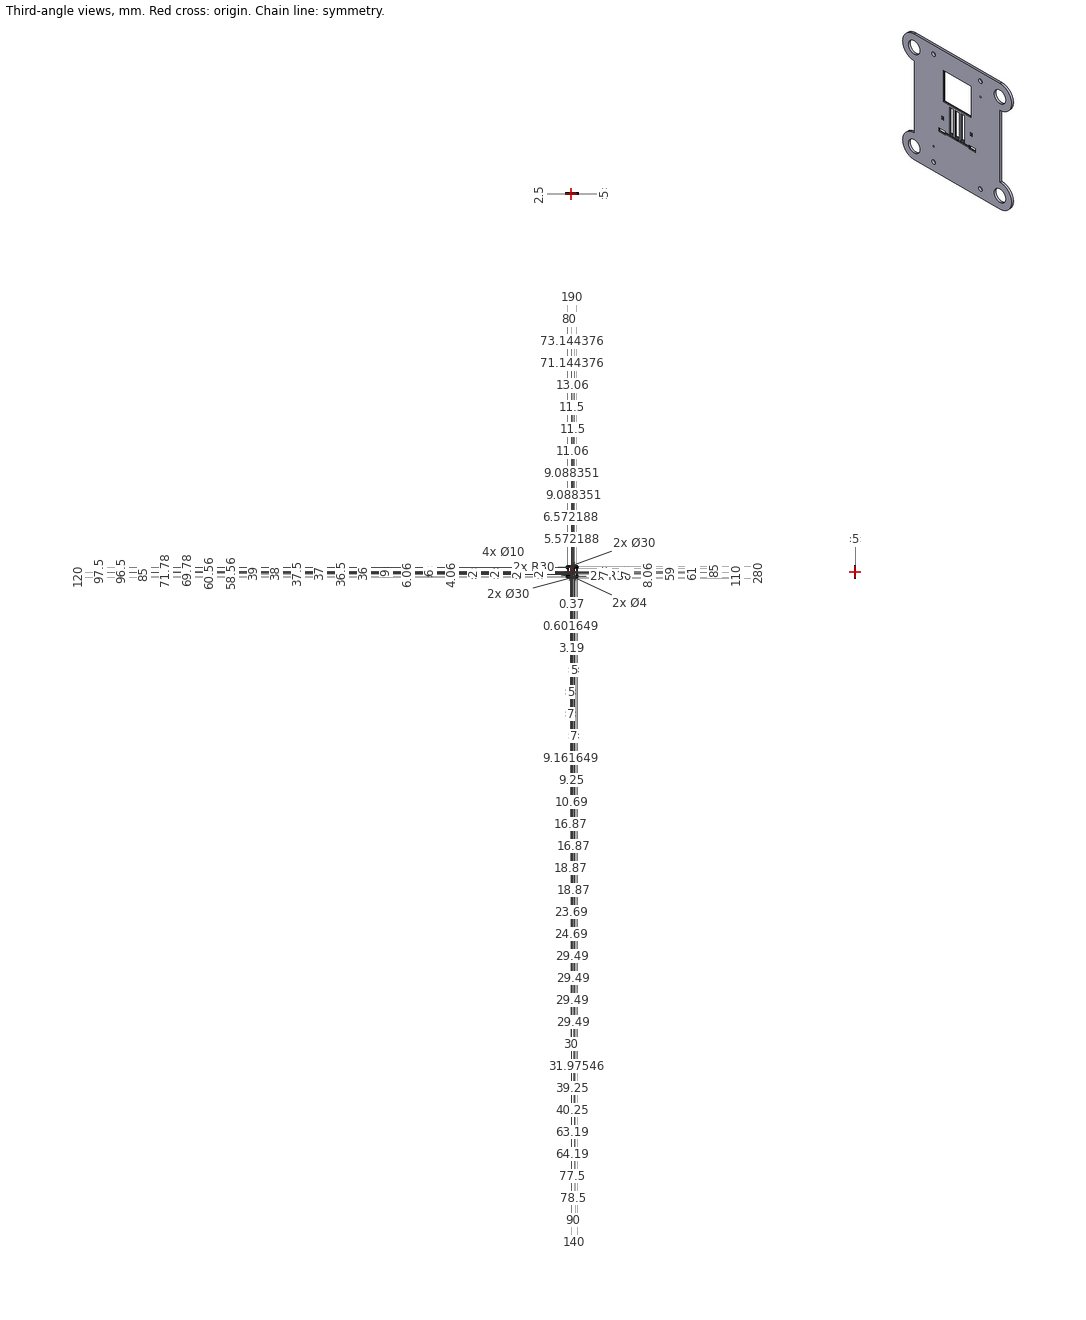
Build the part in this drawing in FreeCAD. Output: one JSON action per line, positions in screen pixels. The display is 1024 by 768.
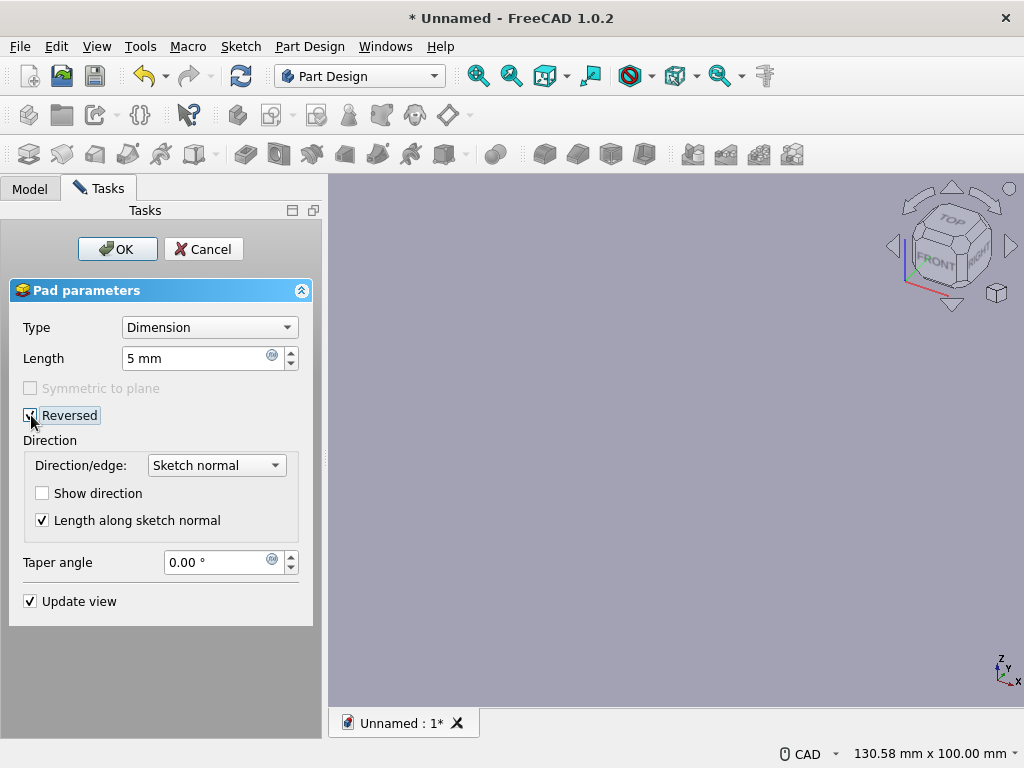
{"action": "left_click", "coordinate": [118, 249]}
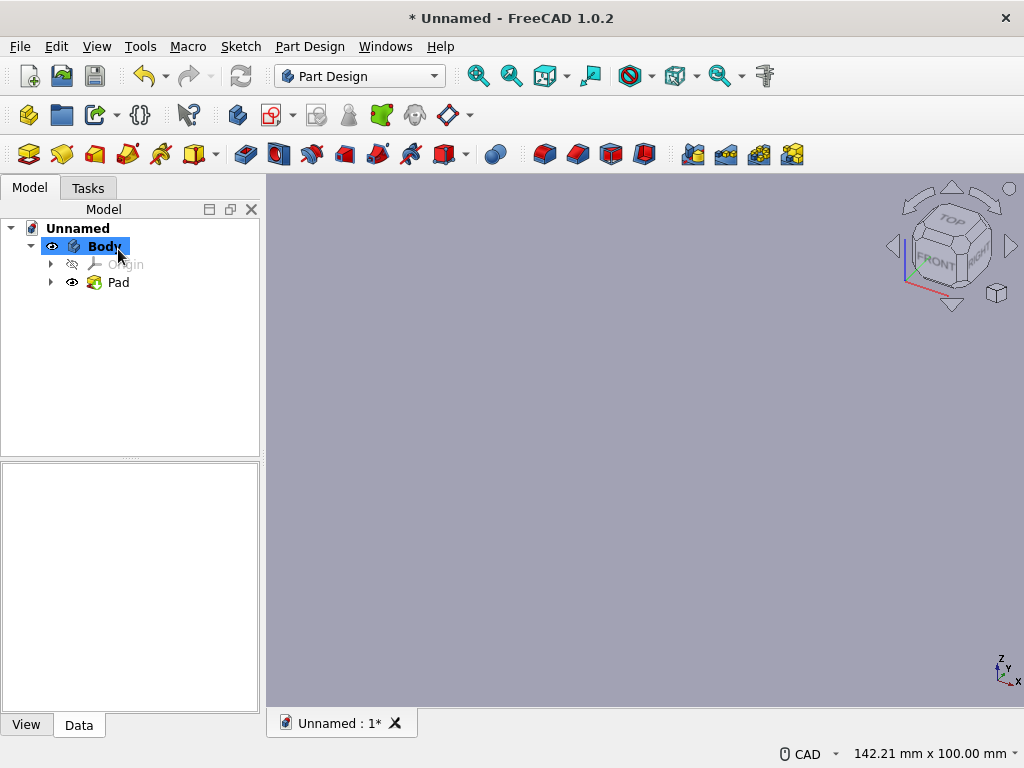
{"action": "left_click", "coordinate": [479, 76]}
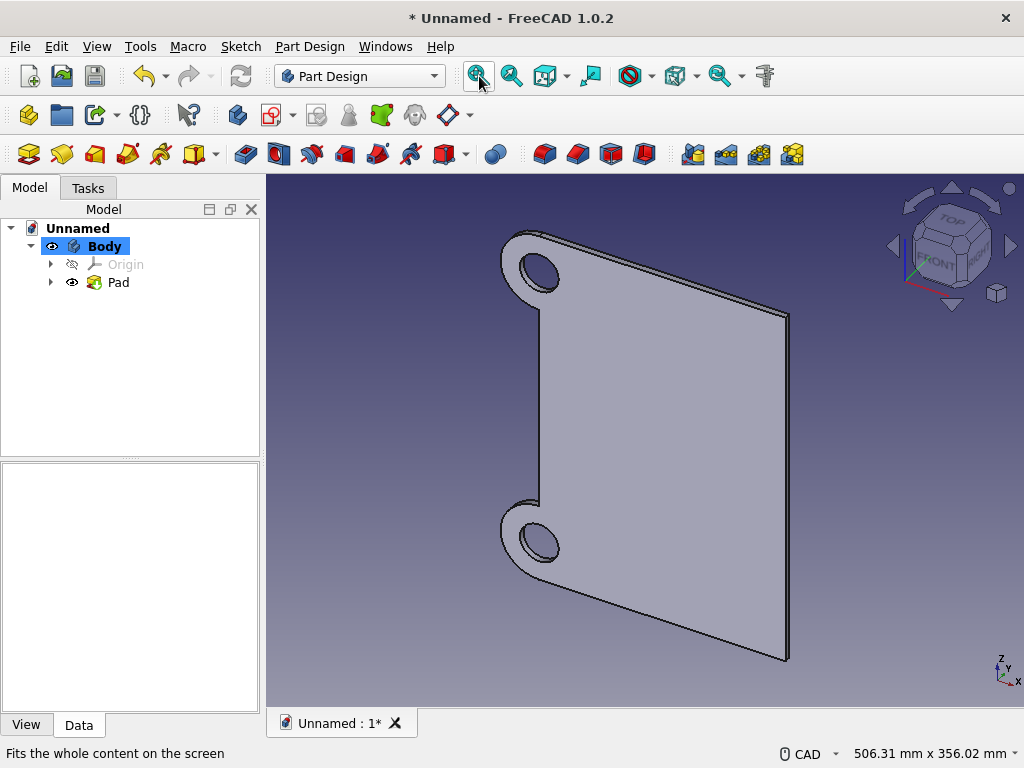
{"action": "key", "text": "4"}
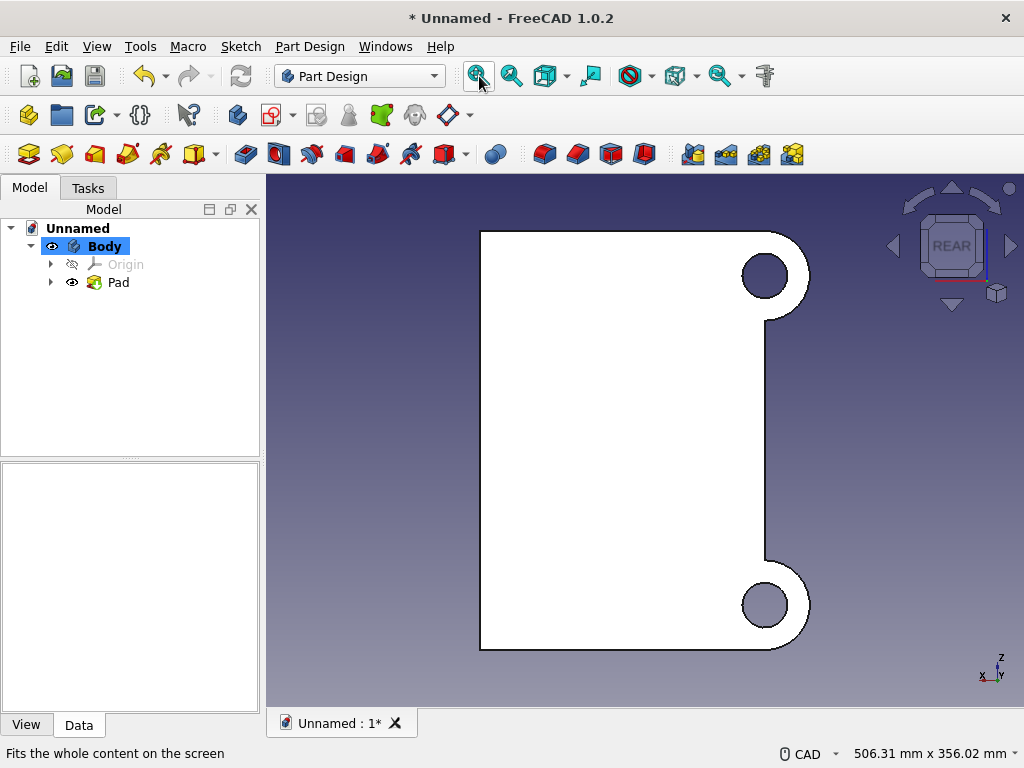
{"action": "left_click", "coordinate": [645, 380]}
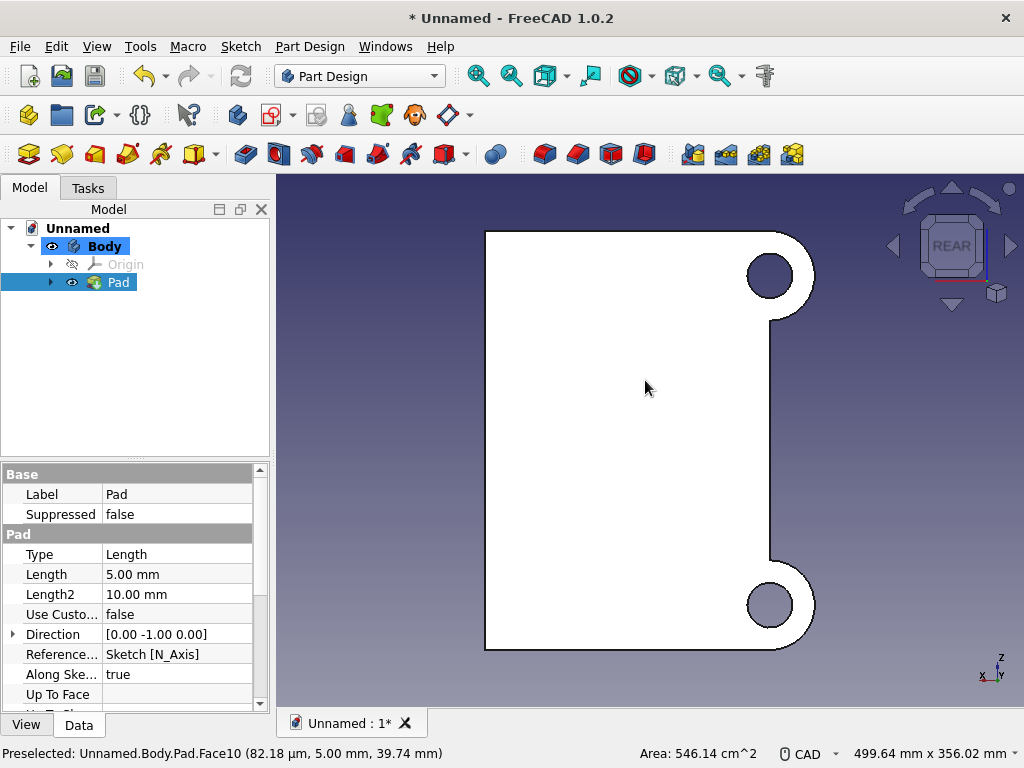
{"action": "left_click", "coordinate": [270, 116]}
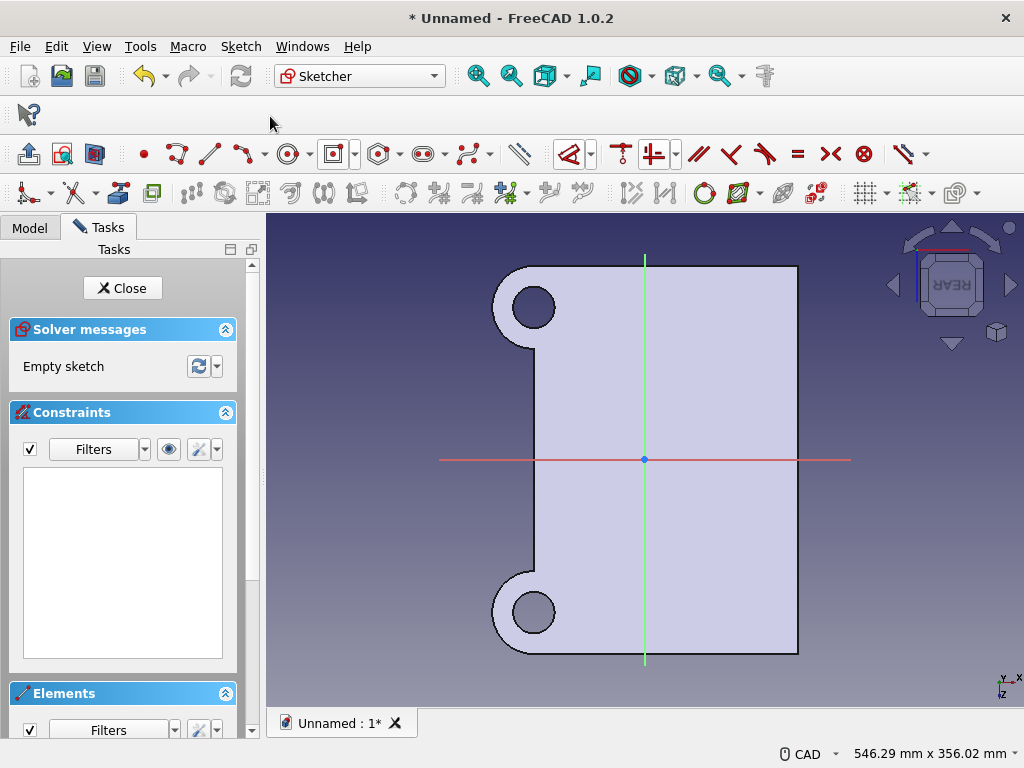
{"action": "scroll", "coordinate": [859, 568], "scroll_direction": "up", "scroll_amount": 2}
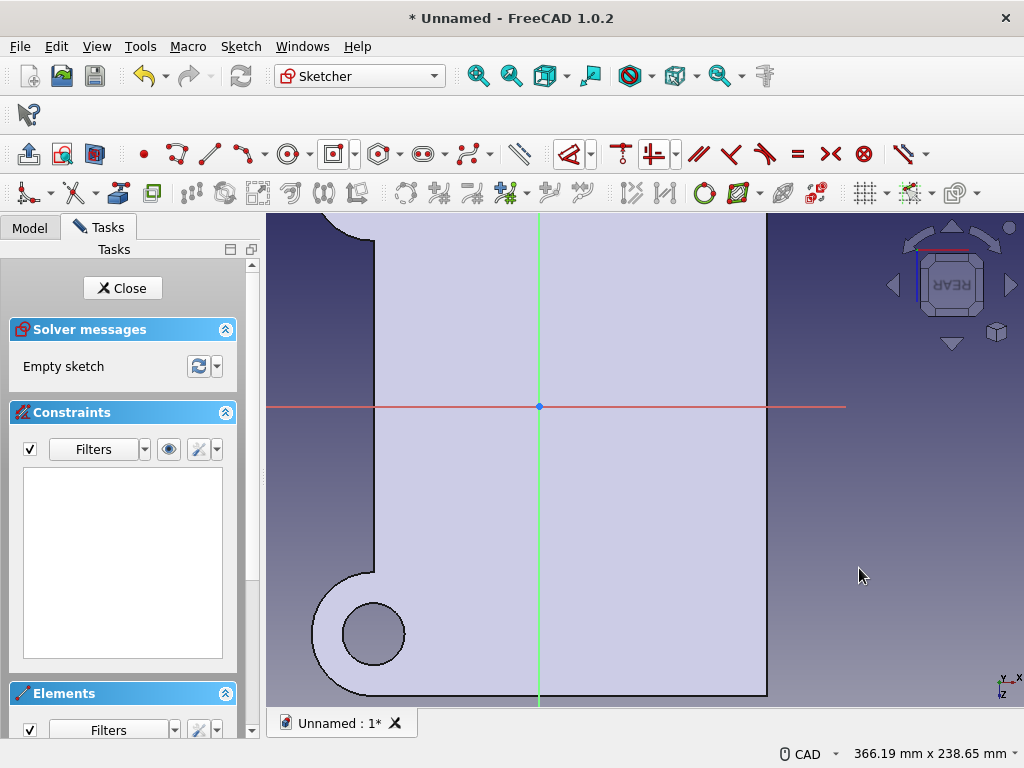
{"action": "key", "text": "g m"}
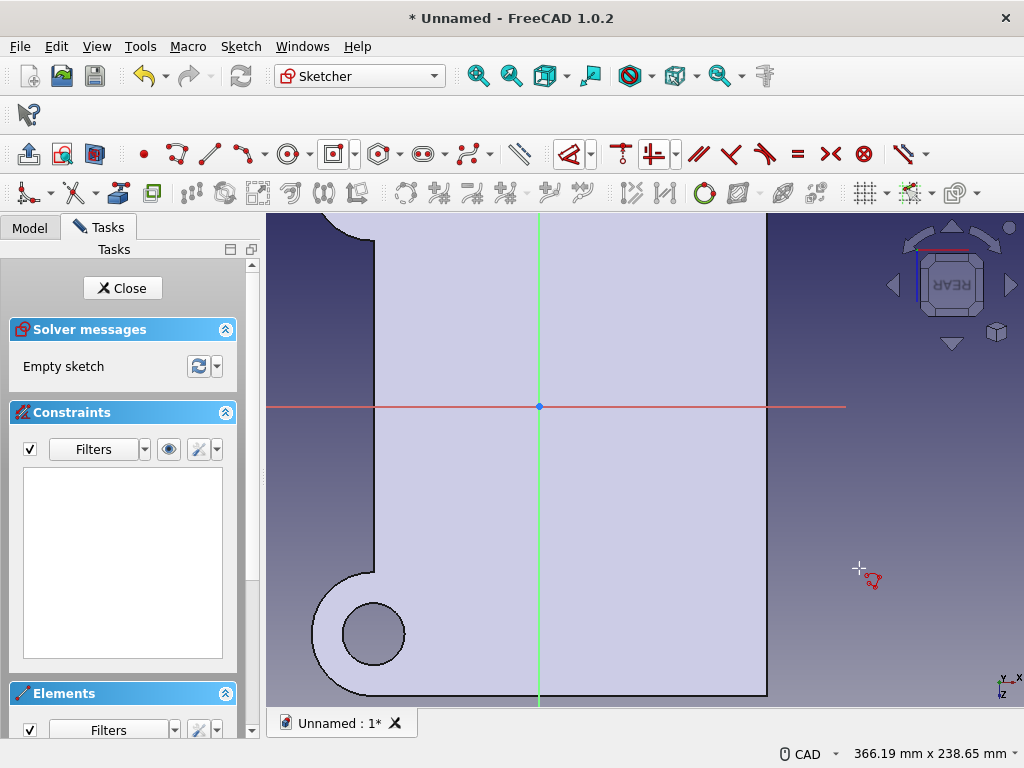
{"action": "scroll", "coordinate": [540, 332], "scroll_direction": "up", "scroll_amount": 16}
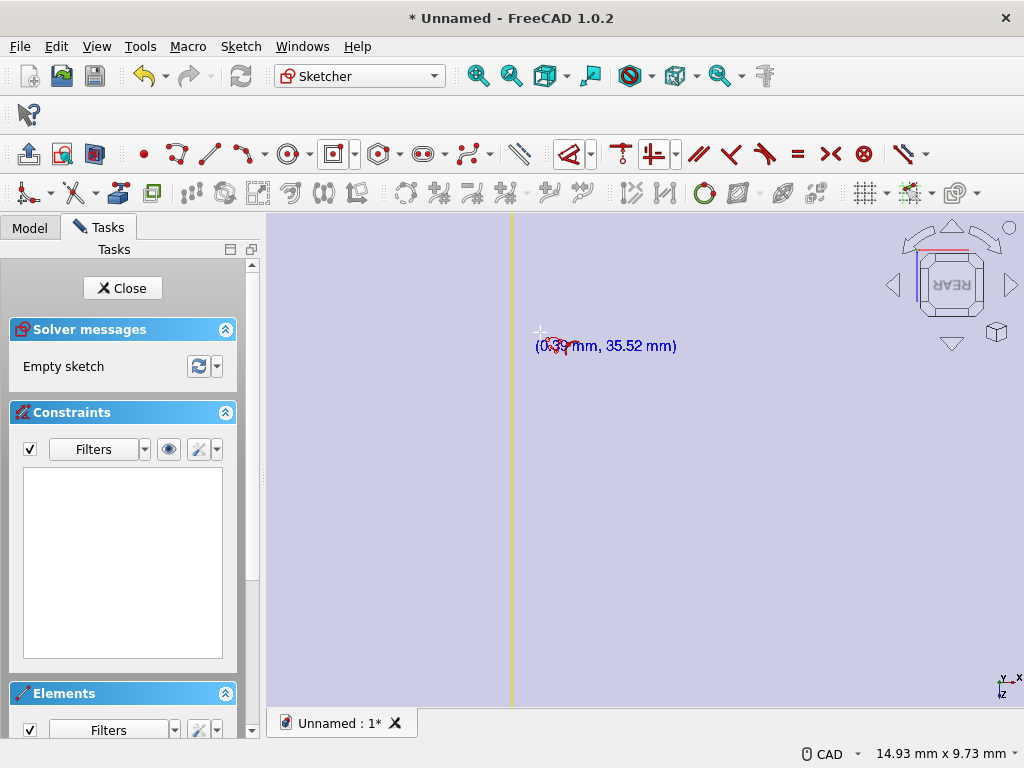
{"action": "left_click", "coordinate": [531, 327]}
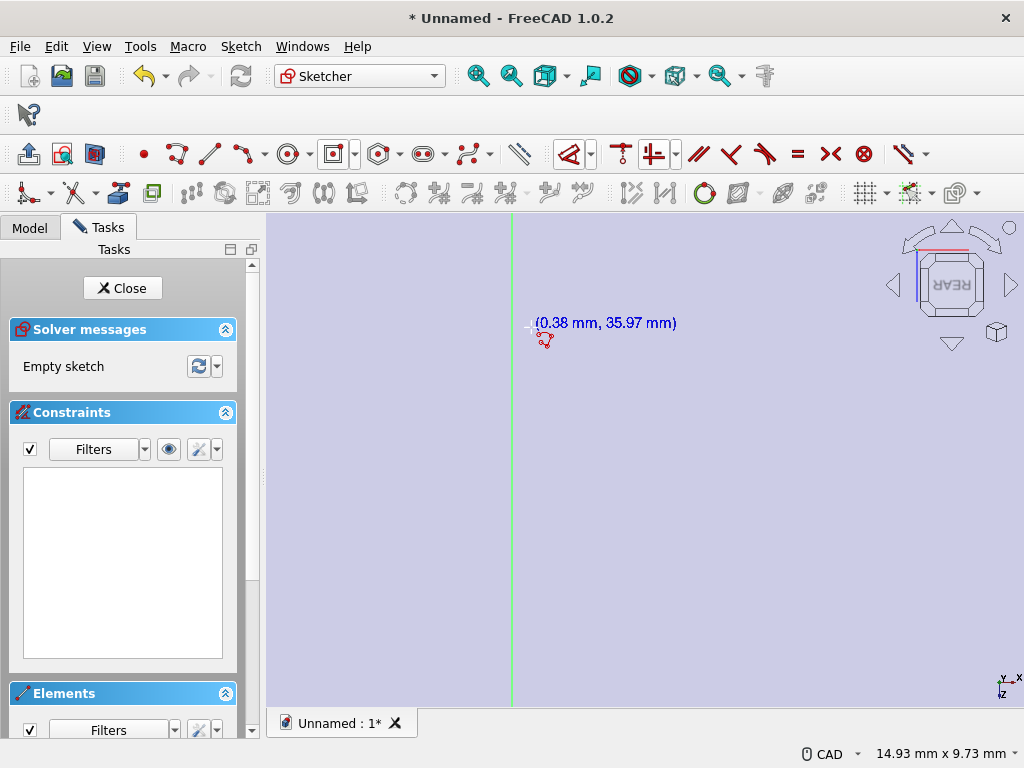
{"action": "scroll", "coordinate": [500, 303], "scroll_direction": "down", "scroll_amount": 15}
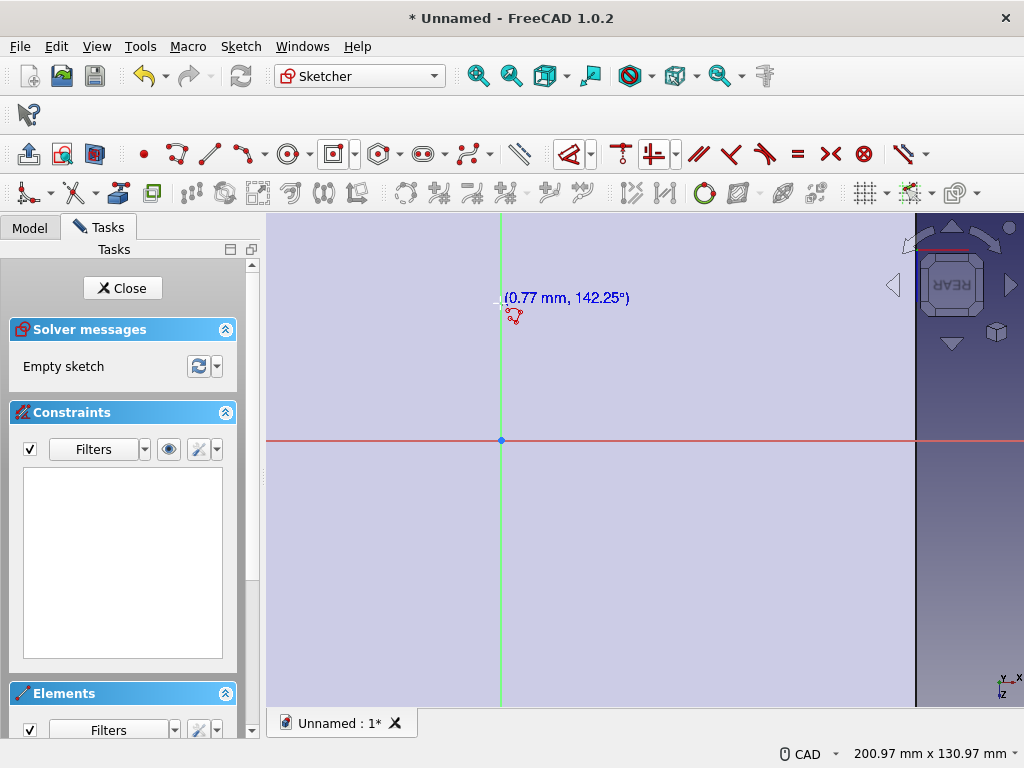
{"action": "scroll", "coordinate": [502, 299], "scroll_direction": "up", "scroll_amount": 15}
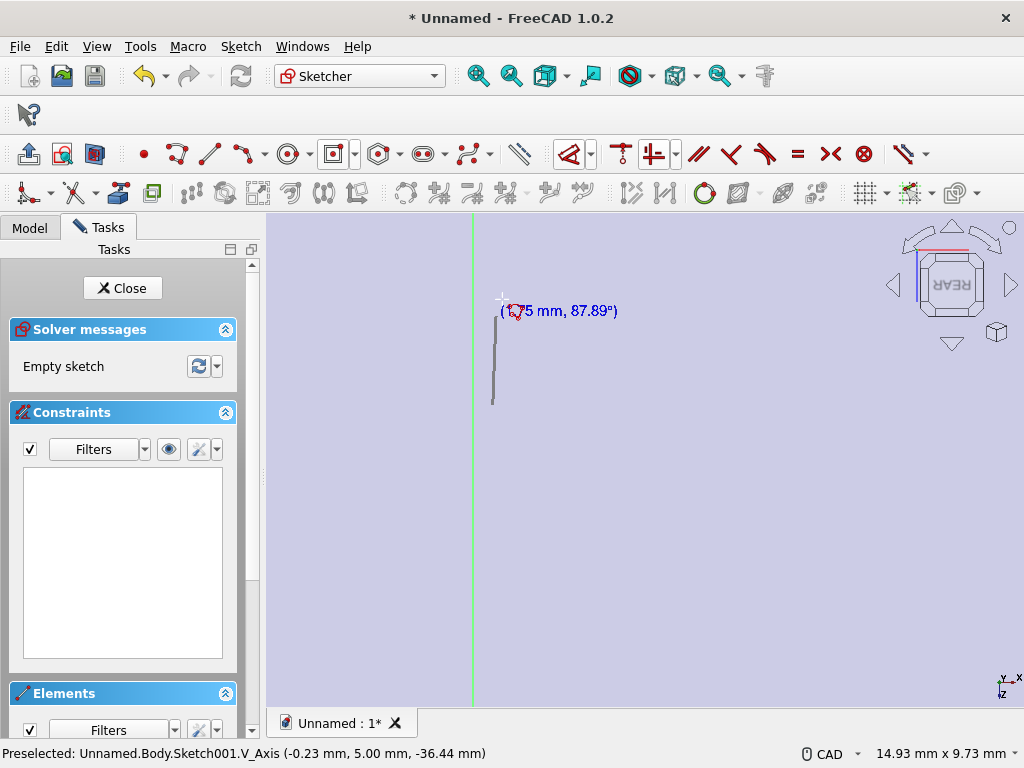
{"action": "left_click", "coordinate": [493, 301]}